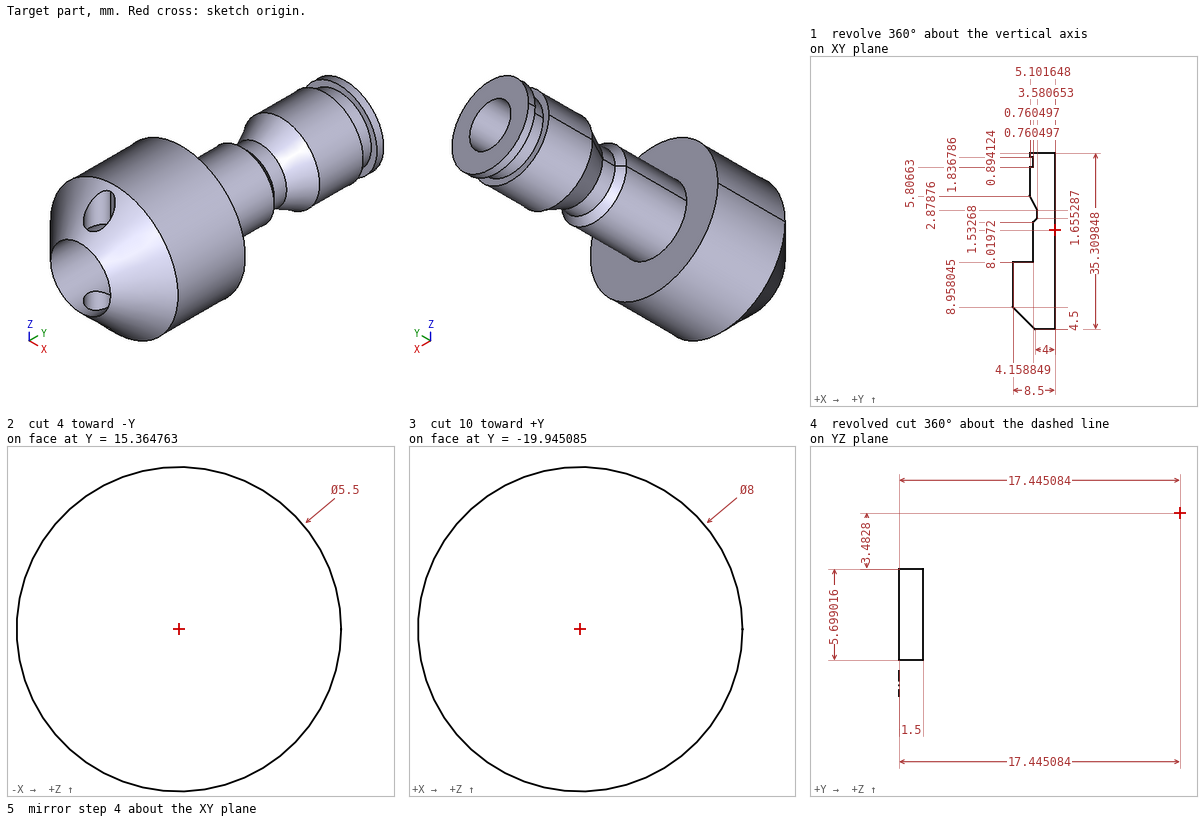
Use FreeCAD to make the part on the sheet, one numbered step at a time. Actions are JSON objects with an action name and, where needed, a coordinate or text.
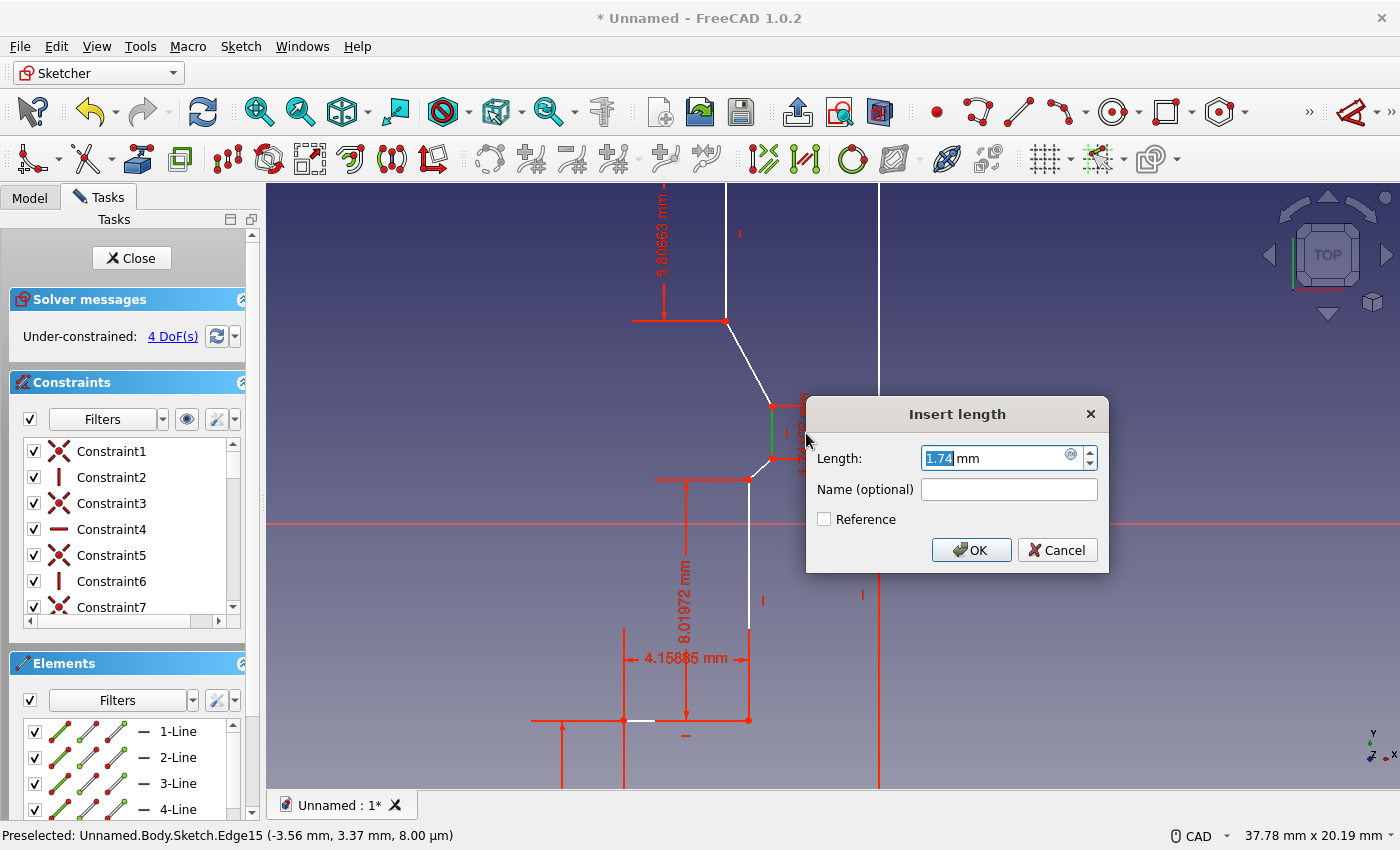
{"action": "type", "text": "1.655287"}
{"action": "key", "text": "Return"}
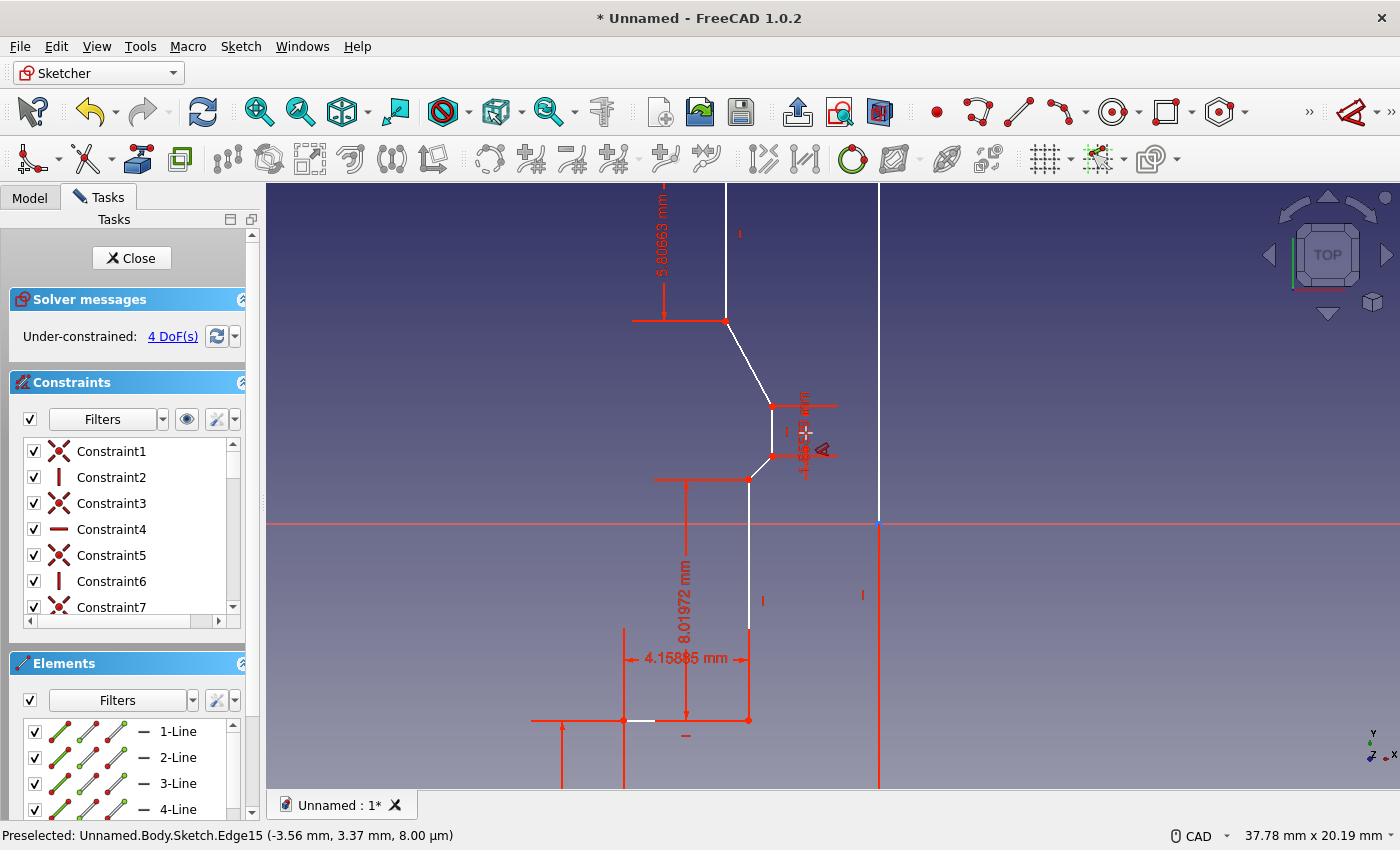
{"action": "left_click", "coordinate": [749, 480]}
{"action": "left_click", "coordinate": [913, 502]}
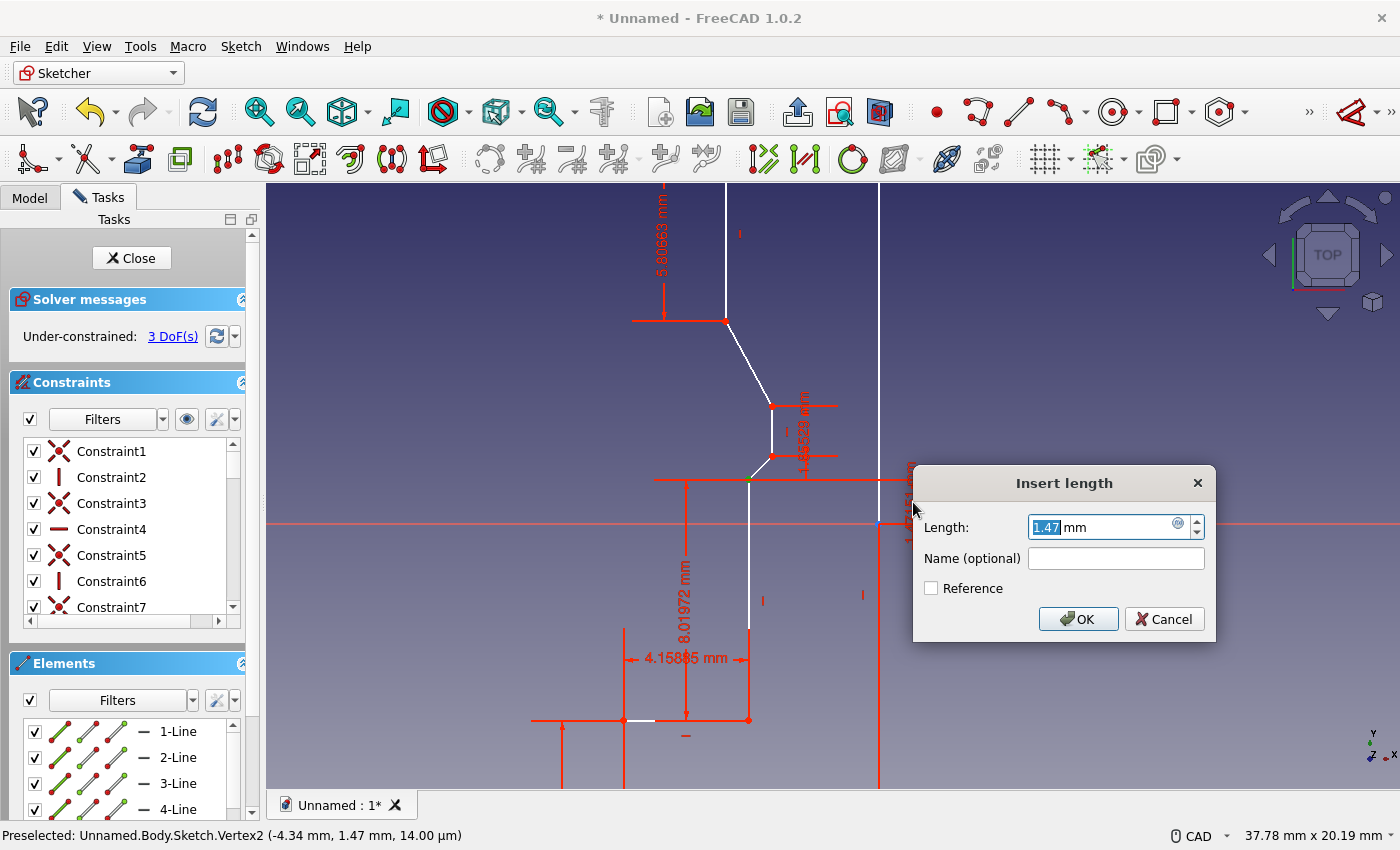
{"action": "type", "text": "1.53268"}
{"action": "key", "text": "Return"}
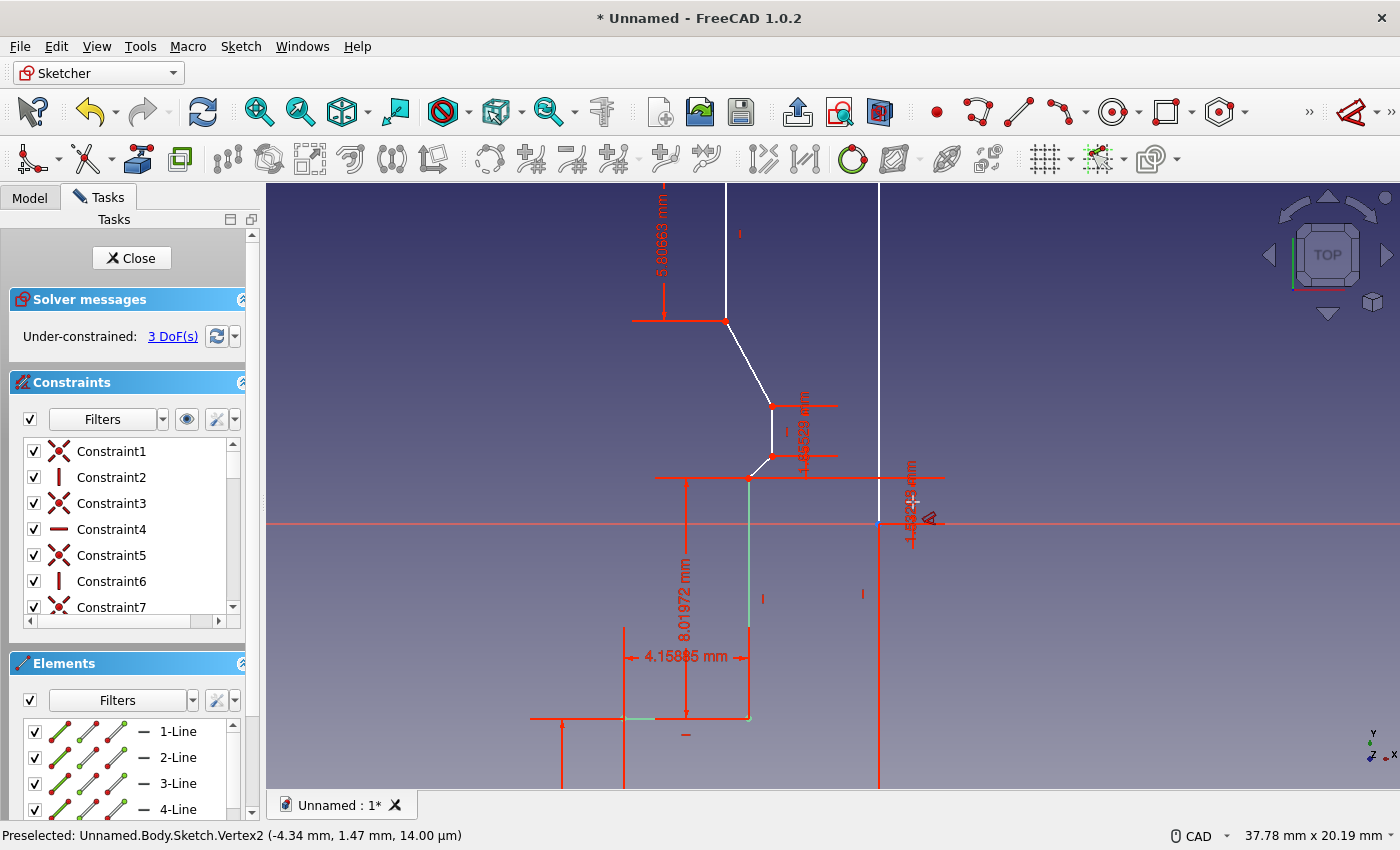
{"action": "left_click", "coordinate": [740, 347]}
{"action": "left_click", "coordinate": [692, 364]}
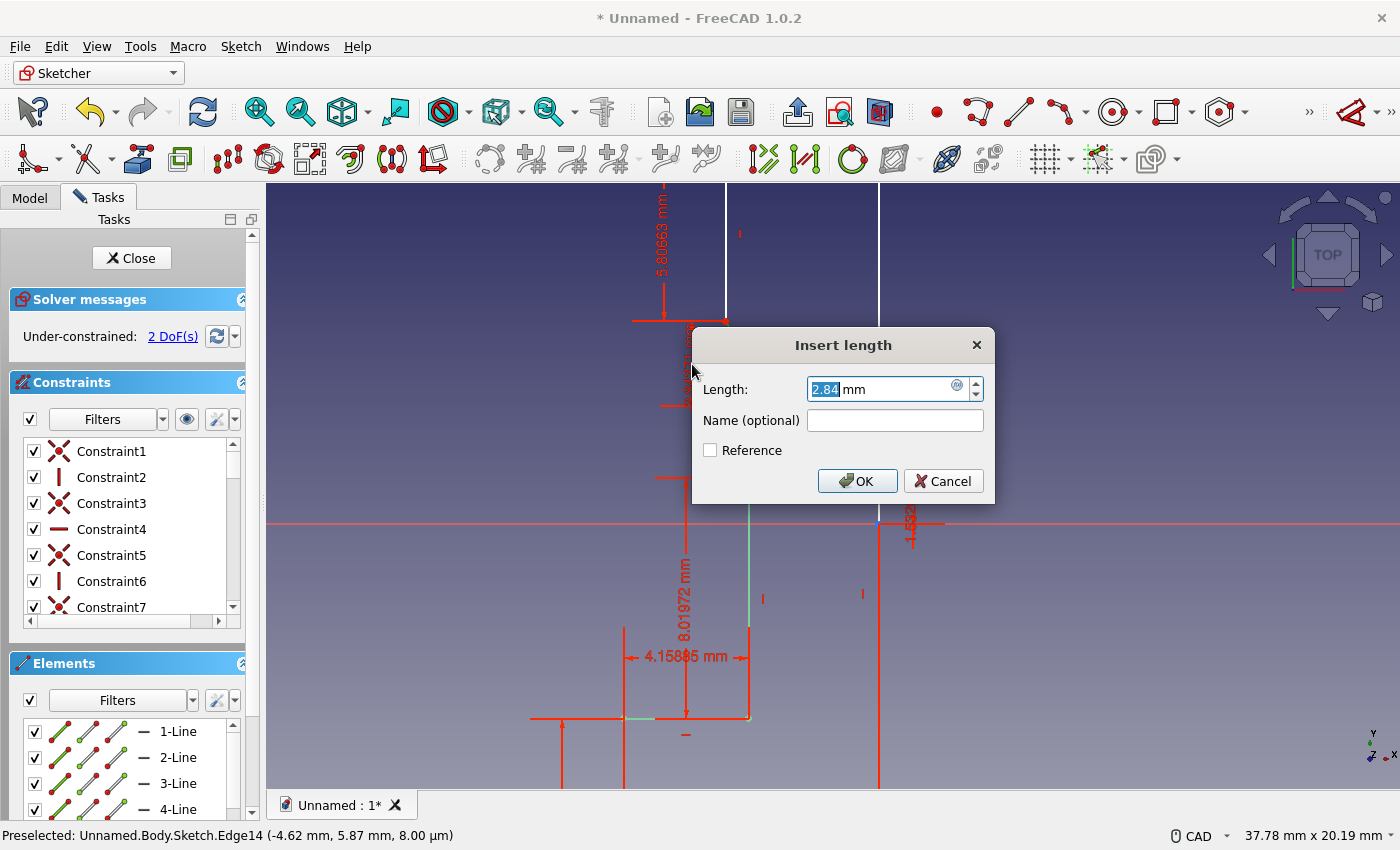
{"action": "type", "text": "2.87876"}
{"action": "key", "text": "Return"}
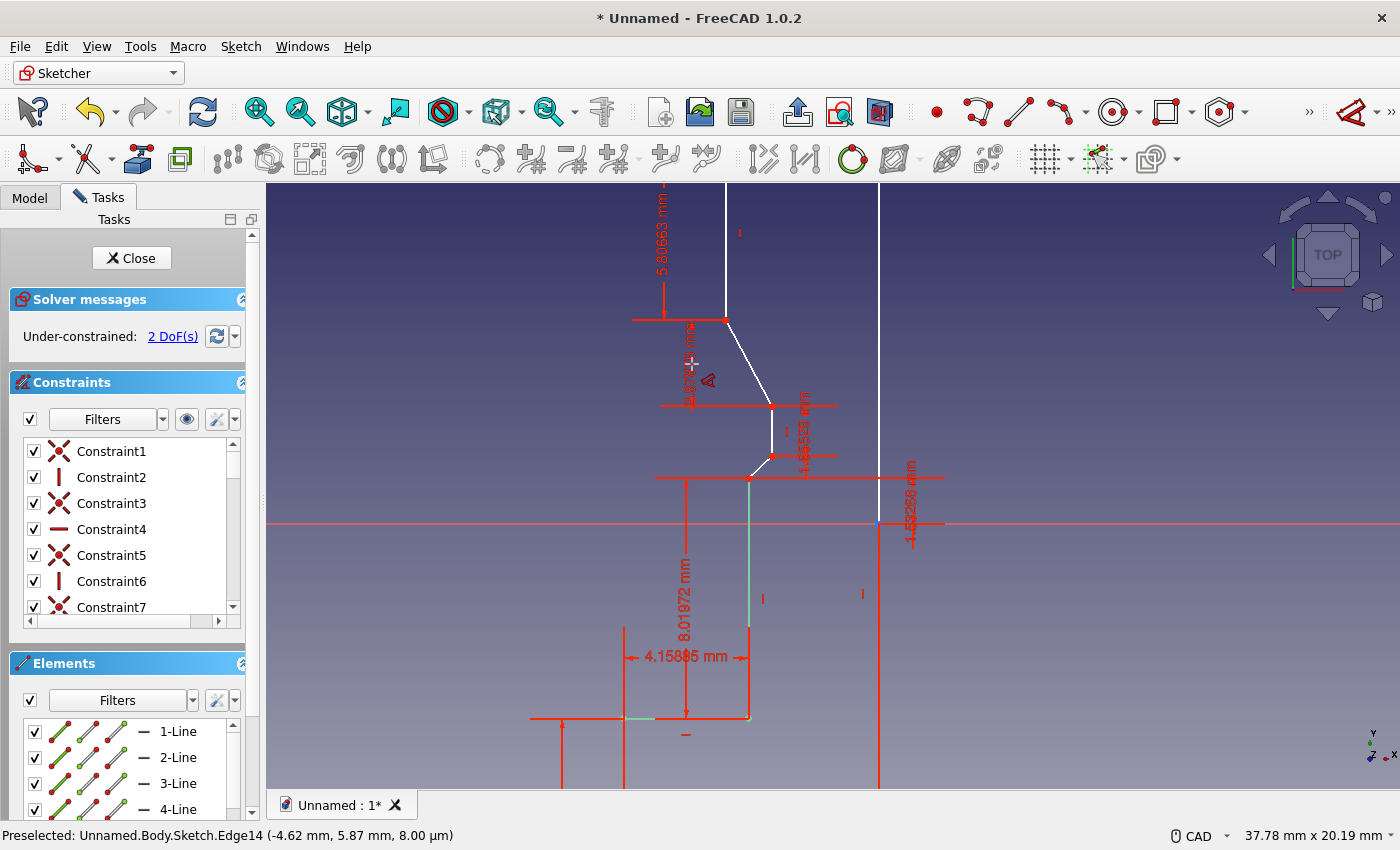
{"action": "left_click", "coordinate": [879, 382]}
{"action": "left_click", "coordinate": [913, 360]}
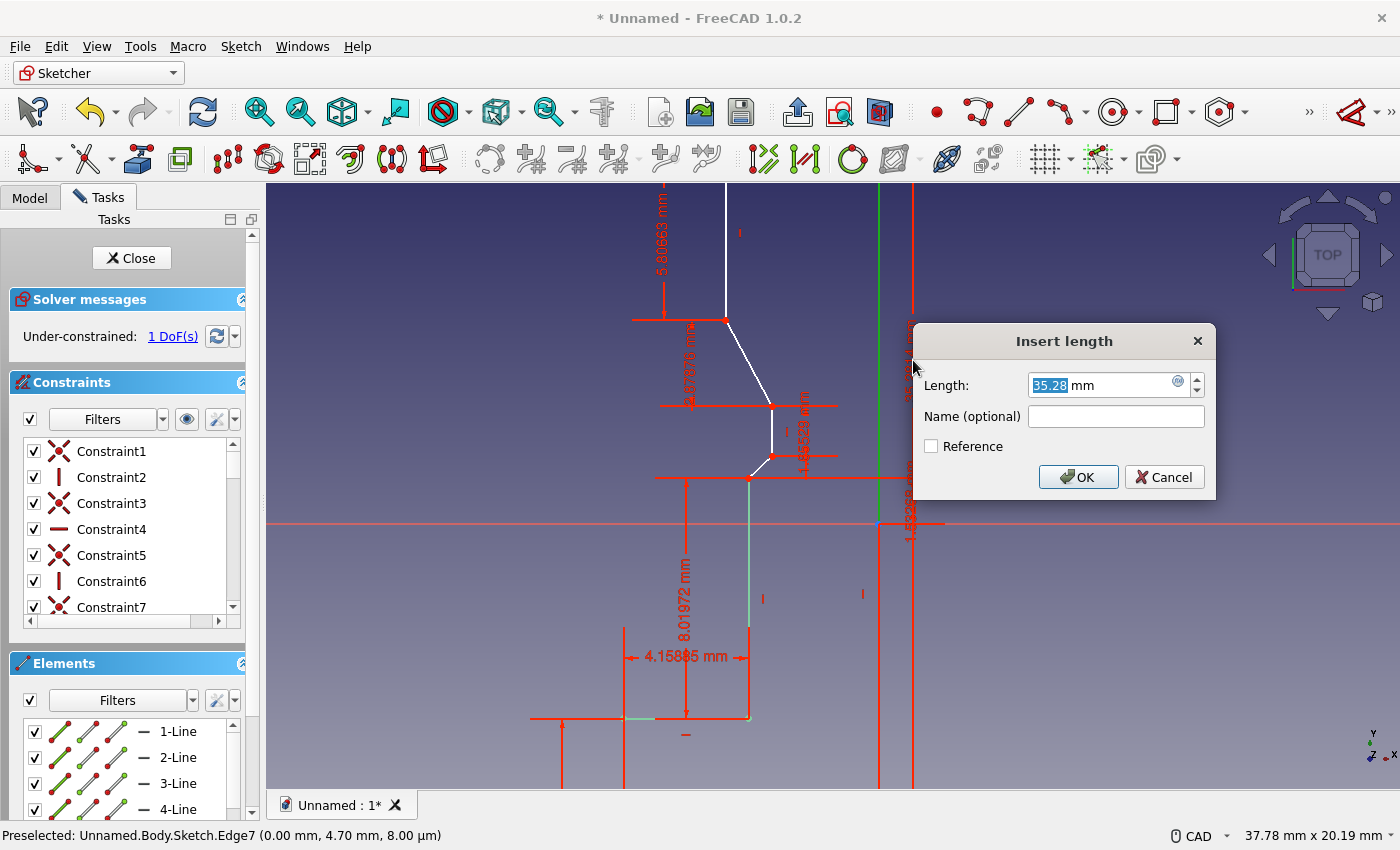
{"action": "type", "text": "35.309848"}
{"action": "key", "text": "Return"}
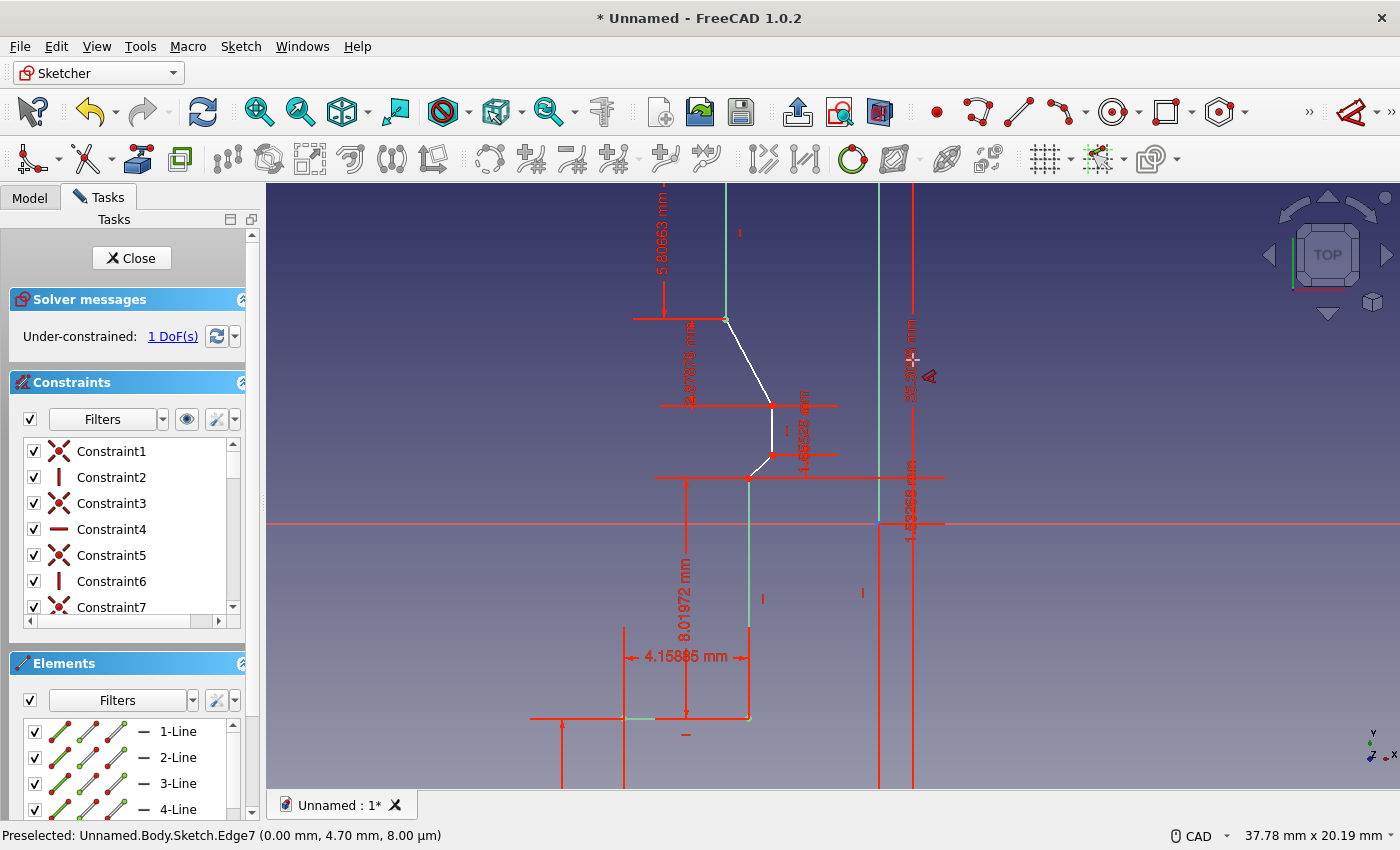
{"action": "left_click", "coordinate": [772, 455]}
{"action": "left_click", "coordinate": [826, 558]}